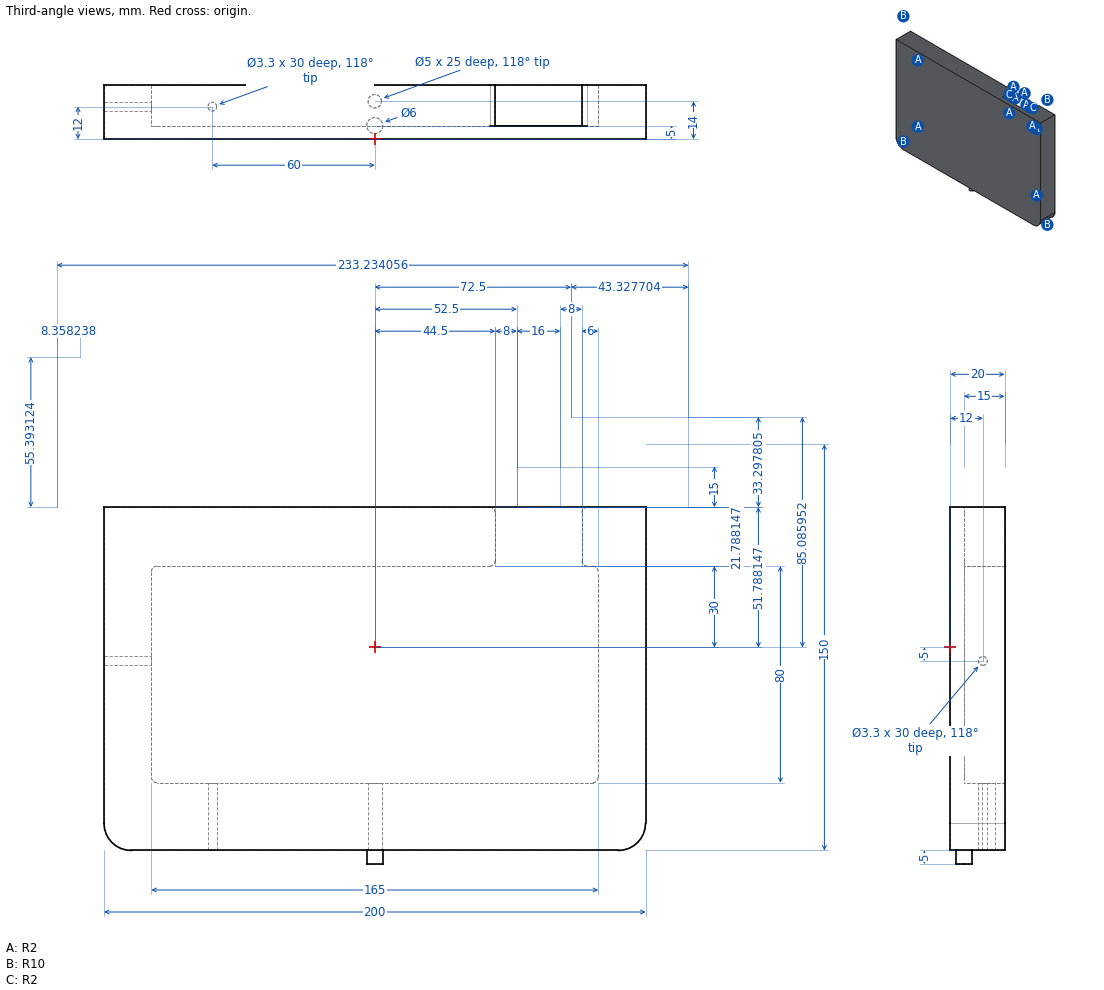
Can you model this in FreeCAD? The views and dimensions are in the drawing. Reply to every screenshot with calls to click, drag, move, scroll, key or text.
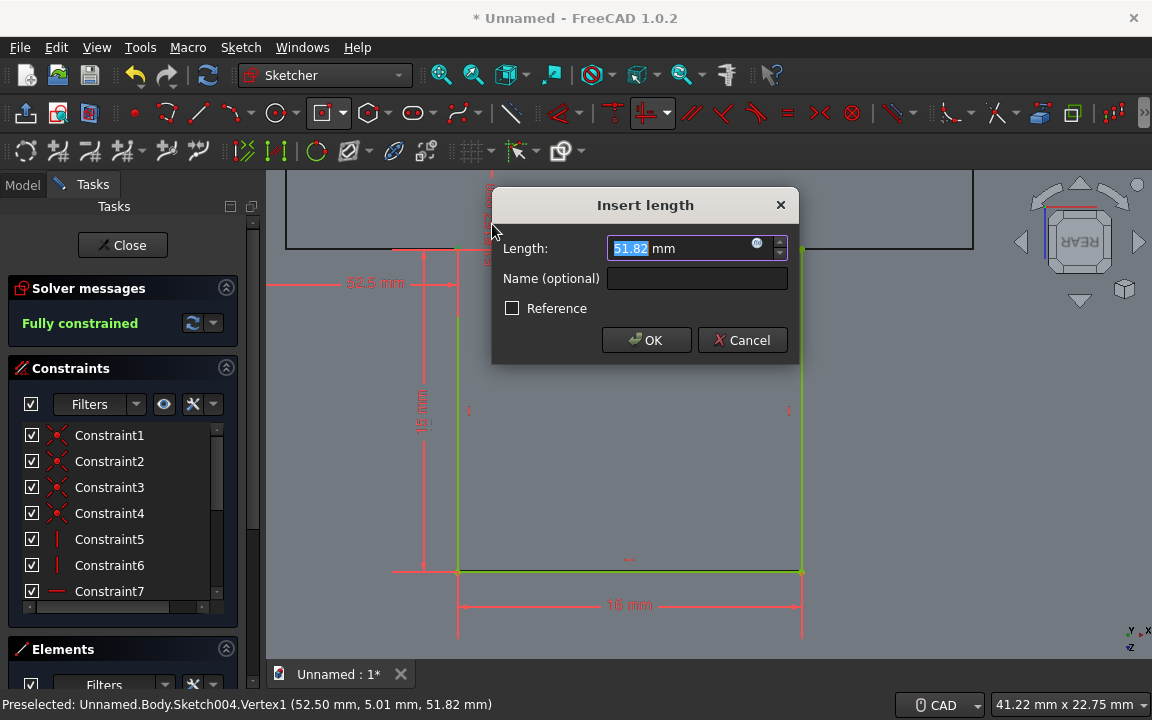
text(51.788147)
key(Return)
key(Escape)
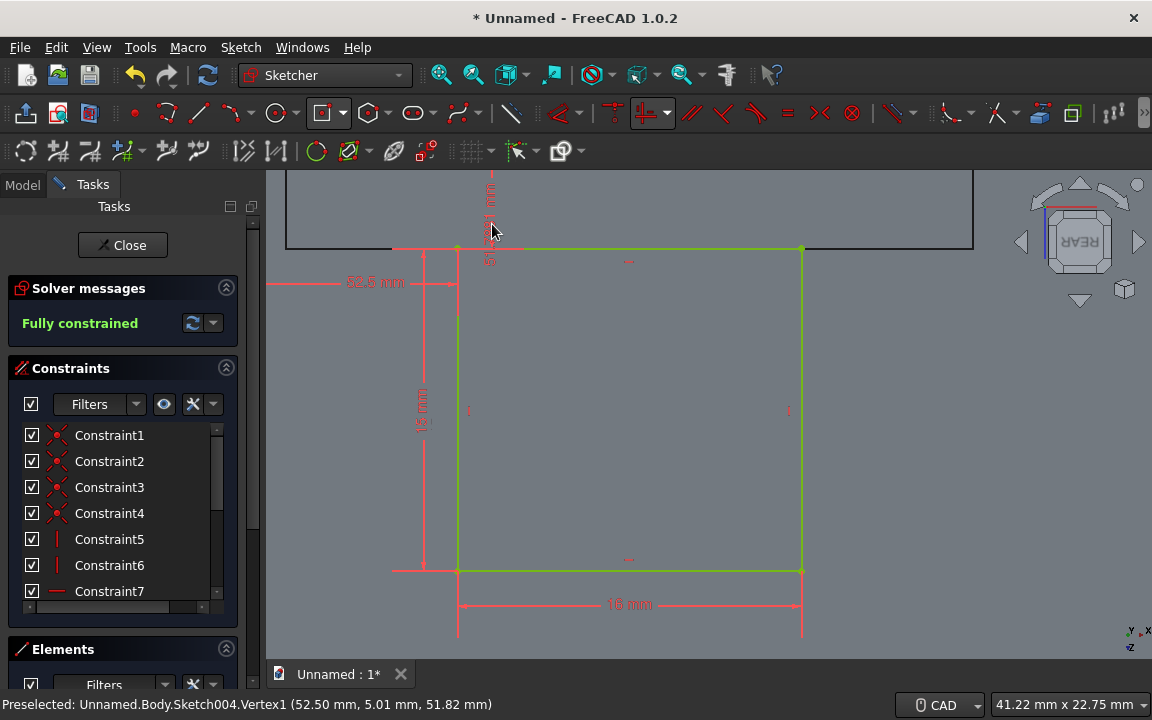
click(123, 245)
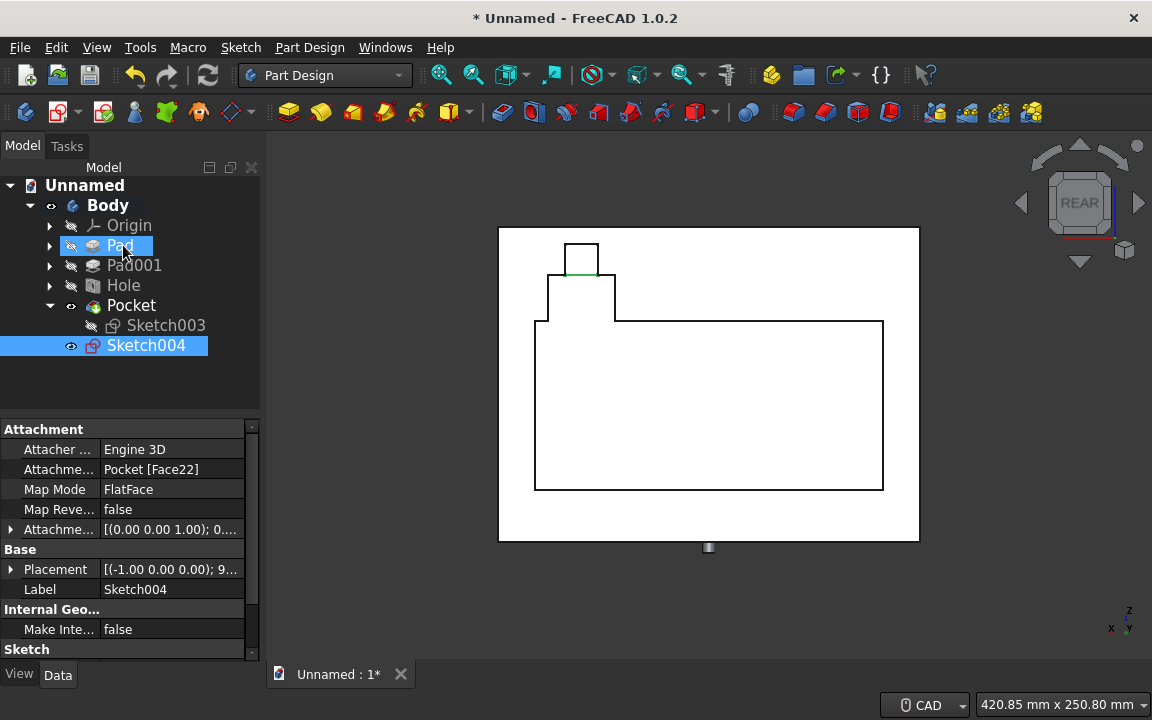
click(504, 112)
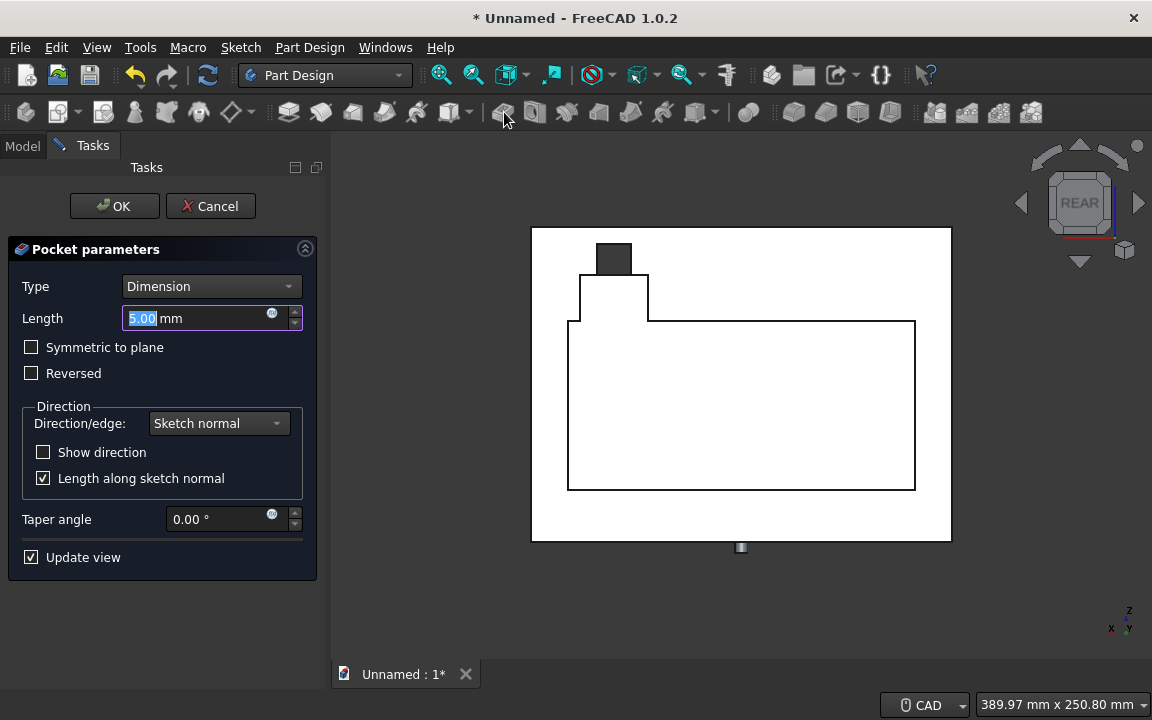
click(212, 286)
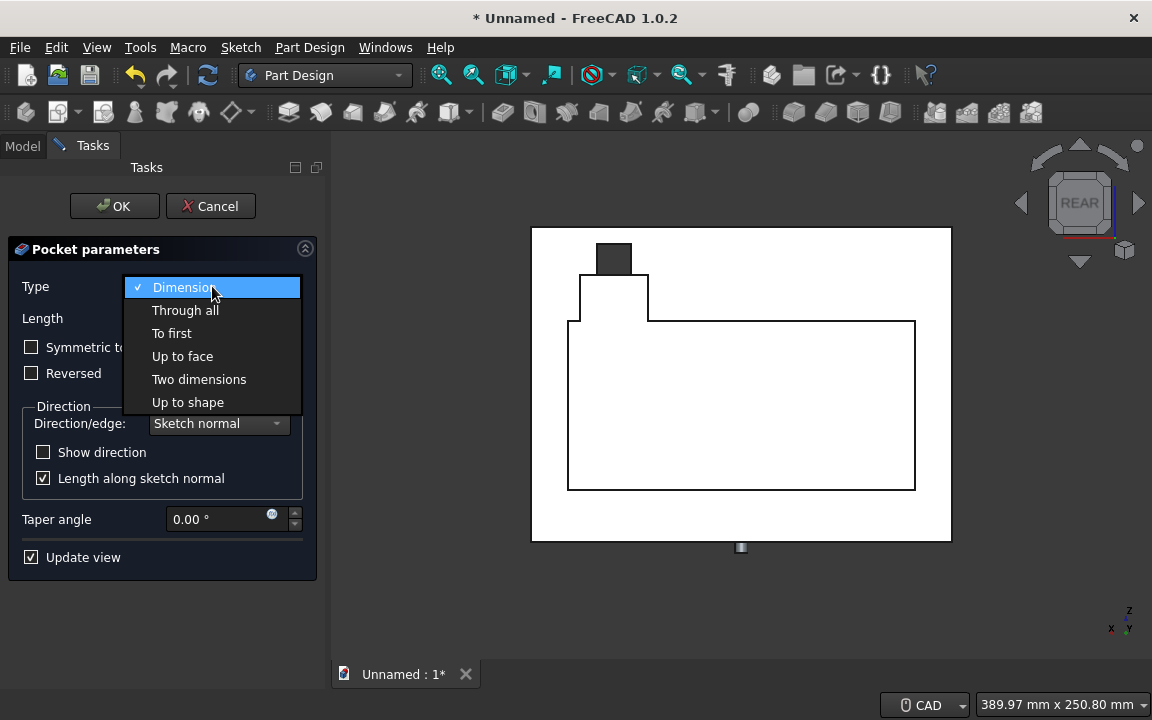
click(212, 310)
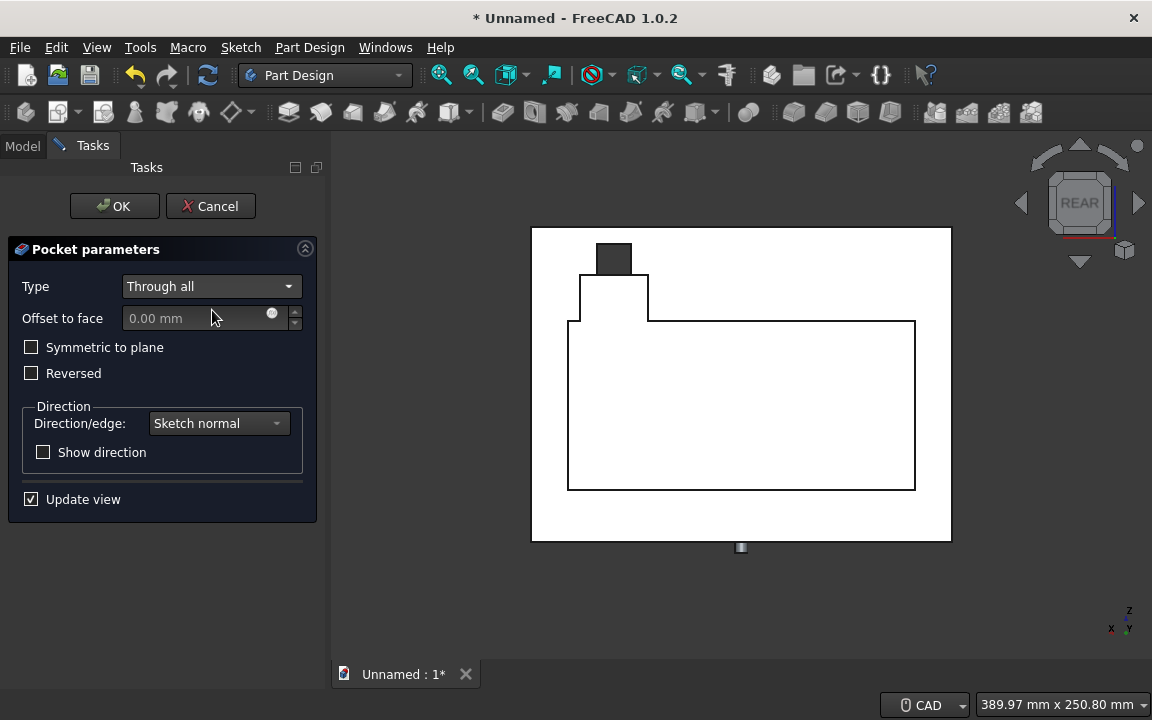
click(115, 206)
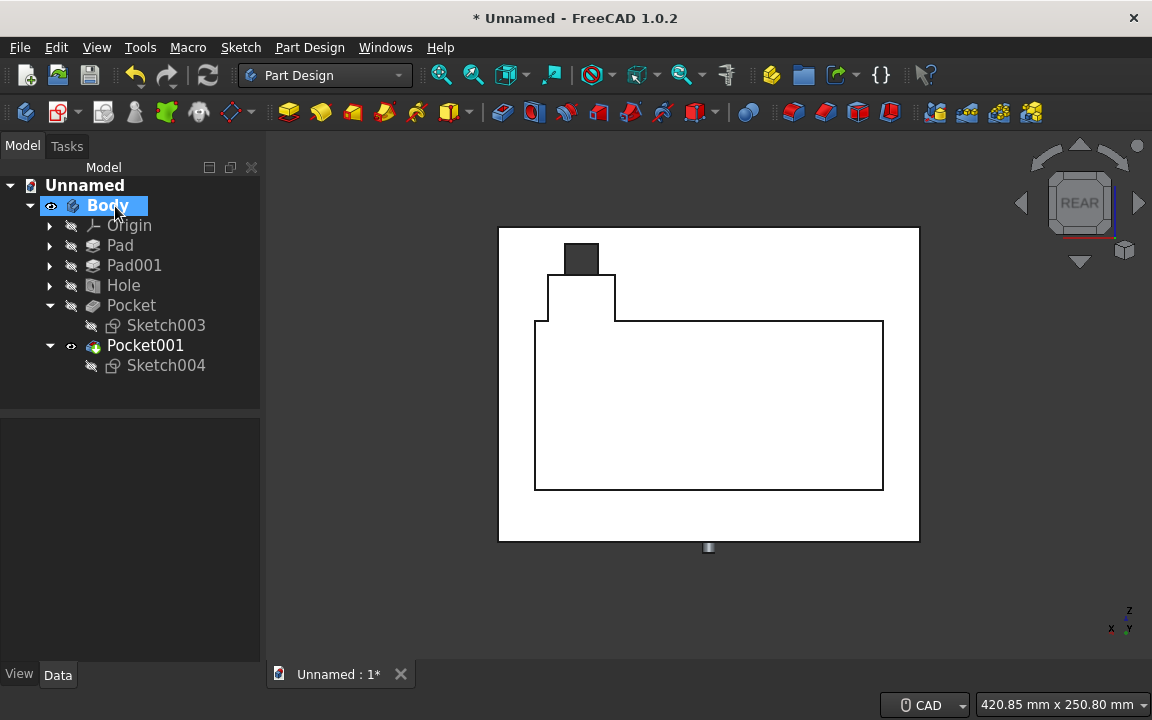
key(0)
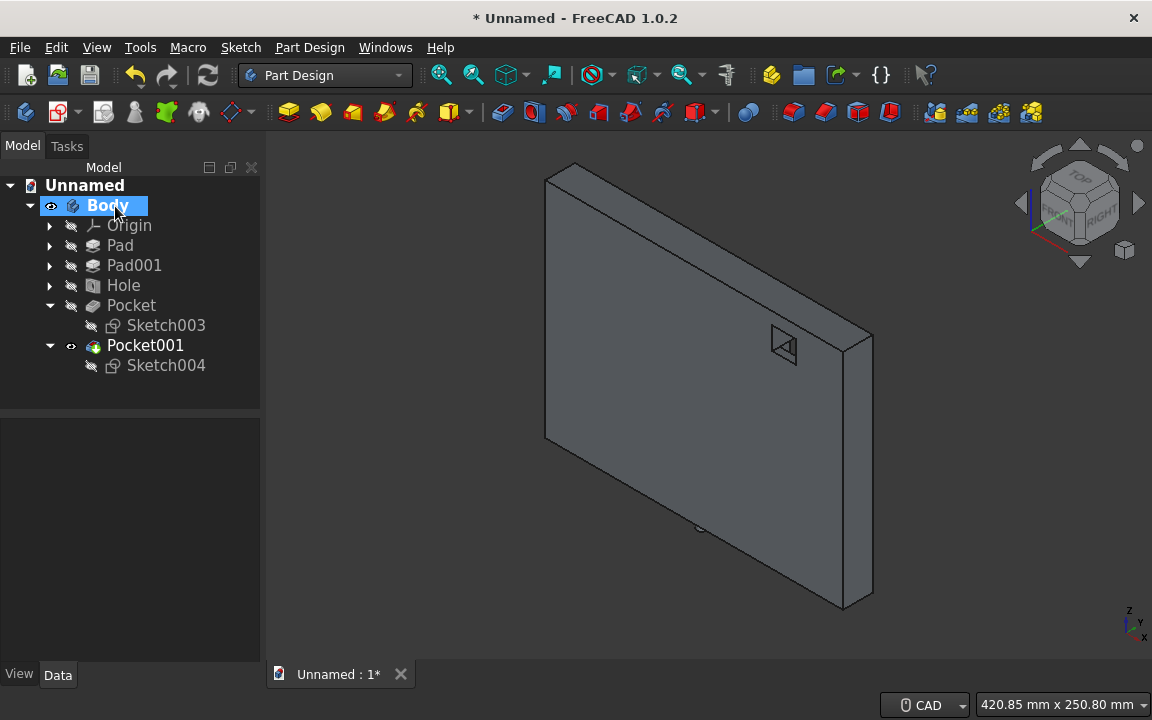
key(2)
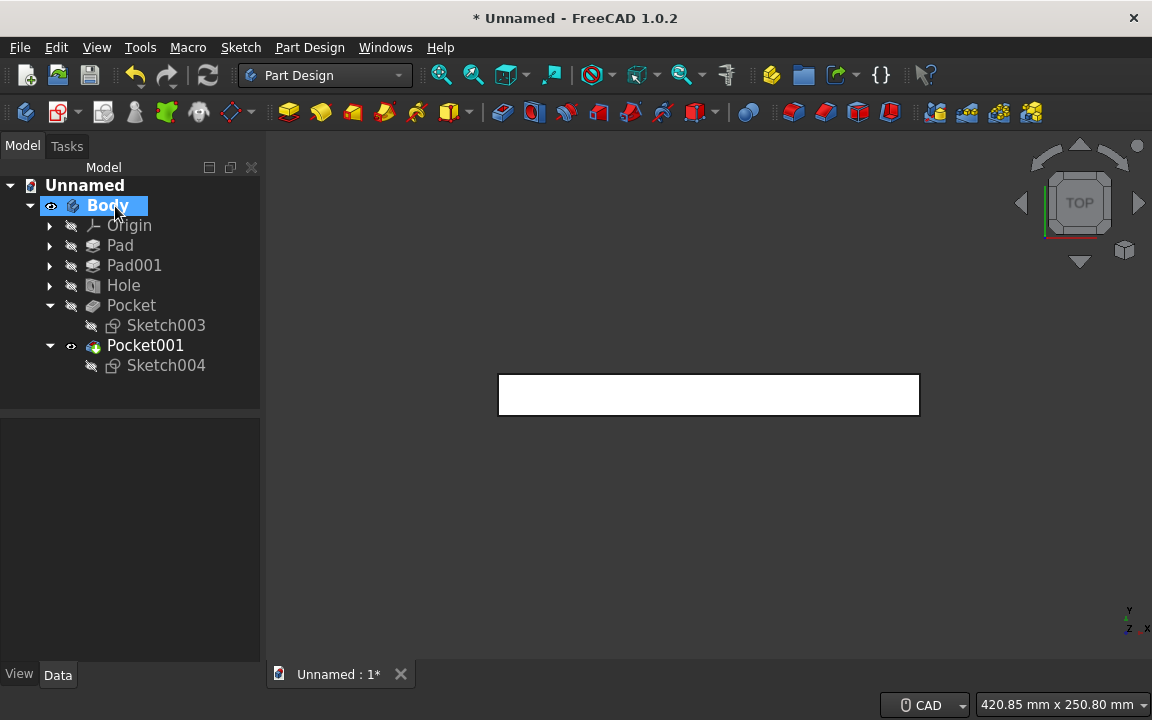
key(1)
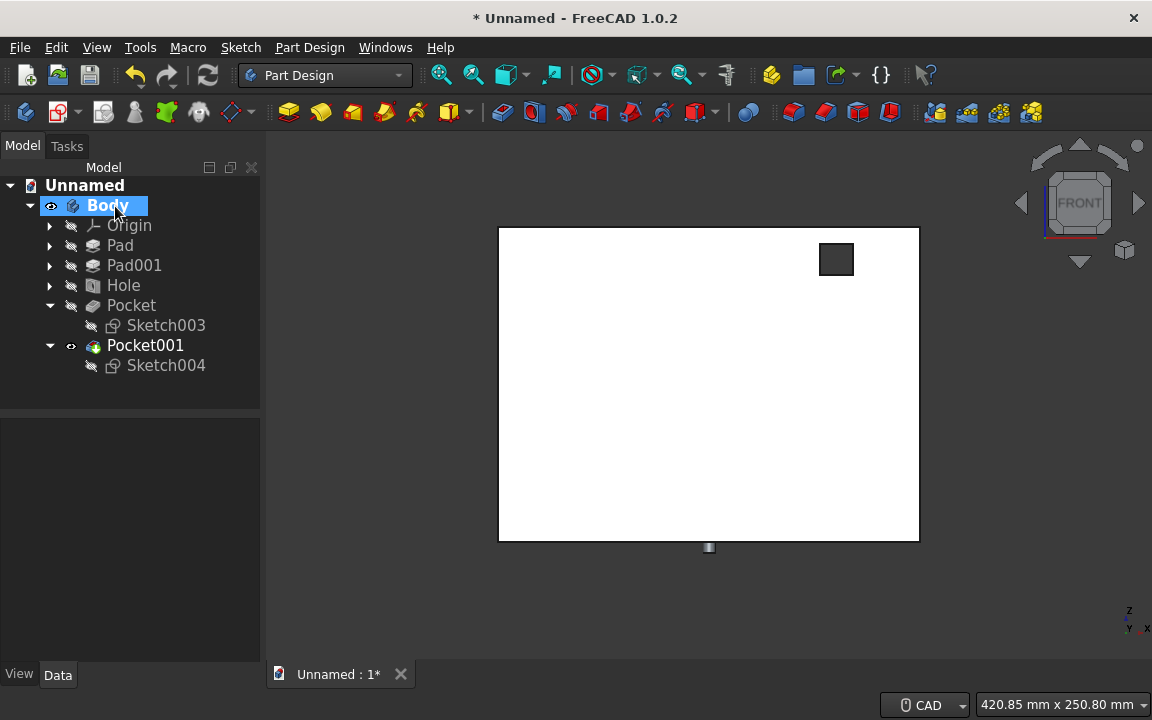
key(3)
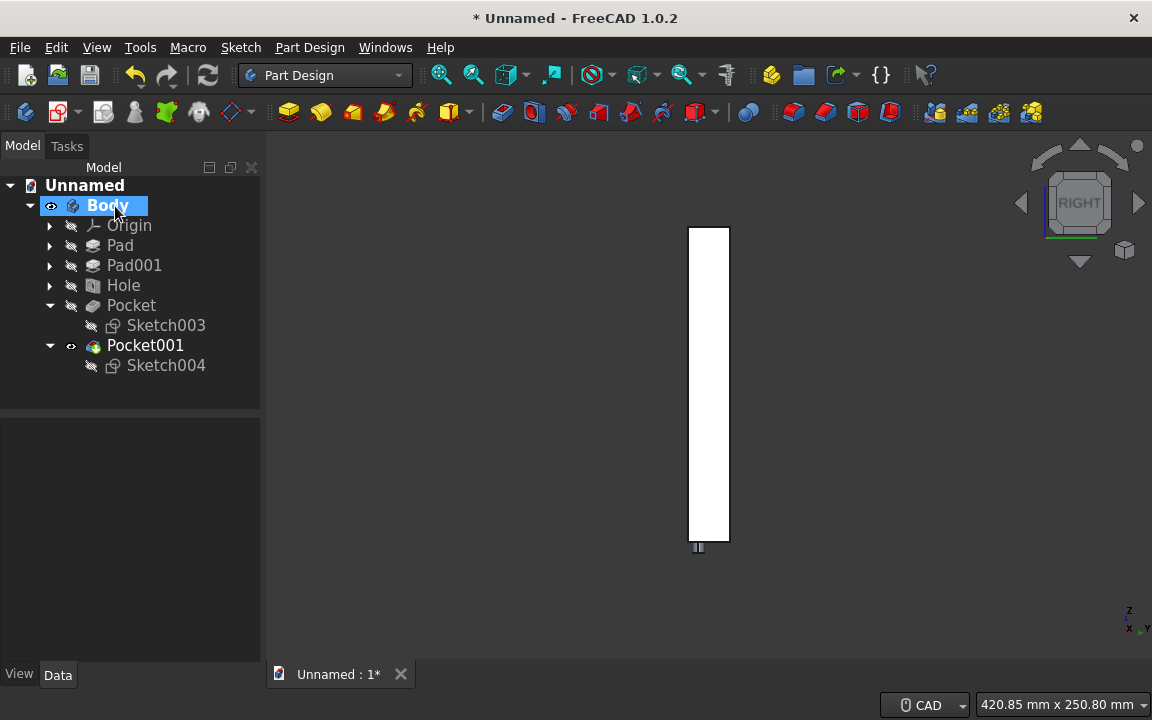
key(5)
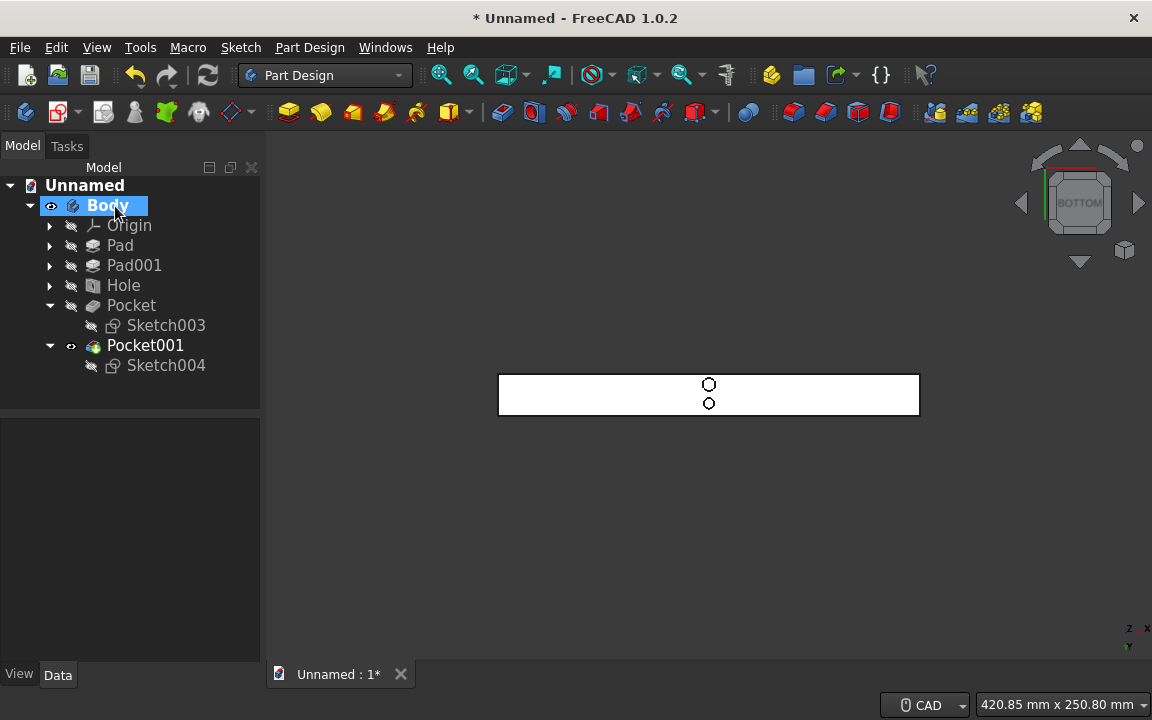
key(4)